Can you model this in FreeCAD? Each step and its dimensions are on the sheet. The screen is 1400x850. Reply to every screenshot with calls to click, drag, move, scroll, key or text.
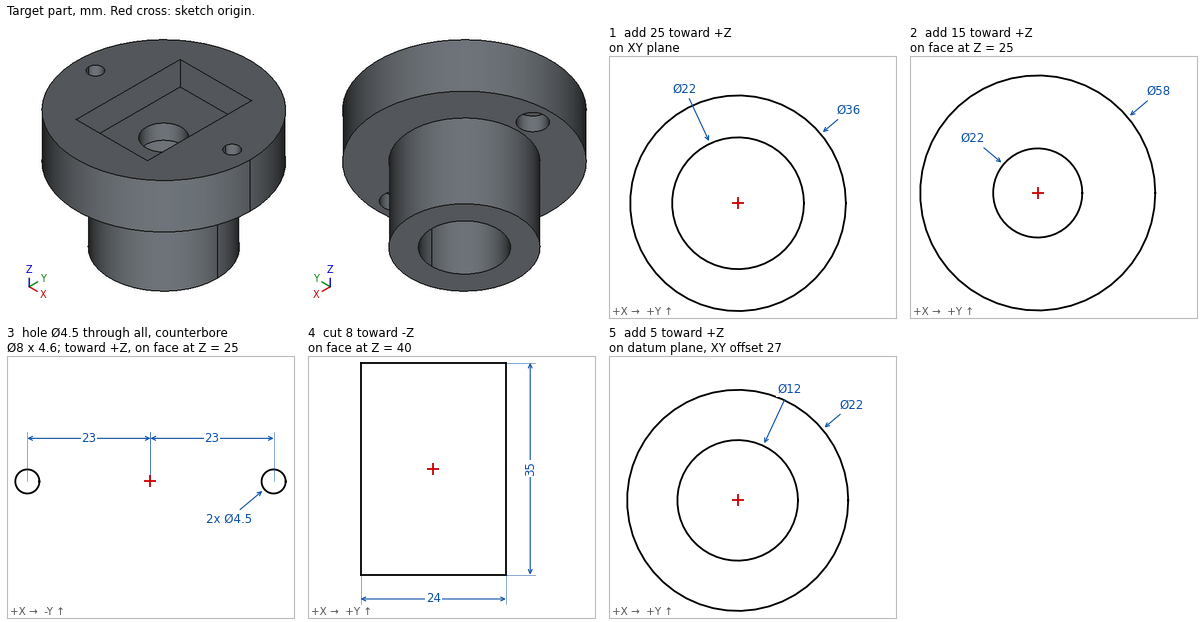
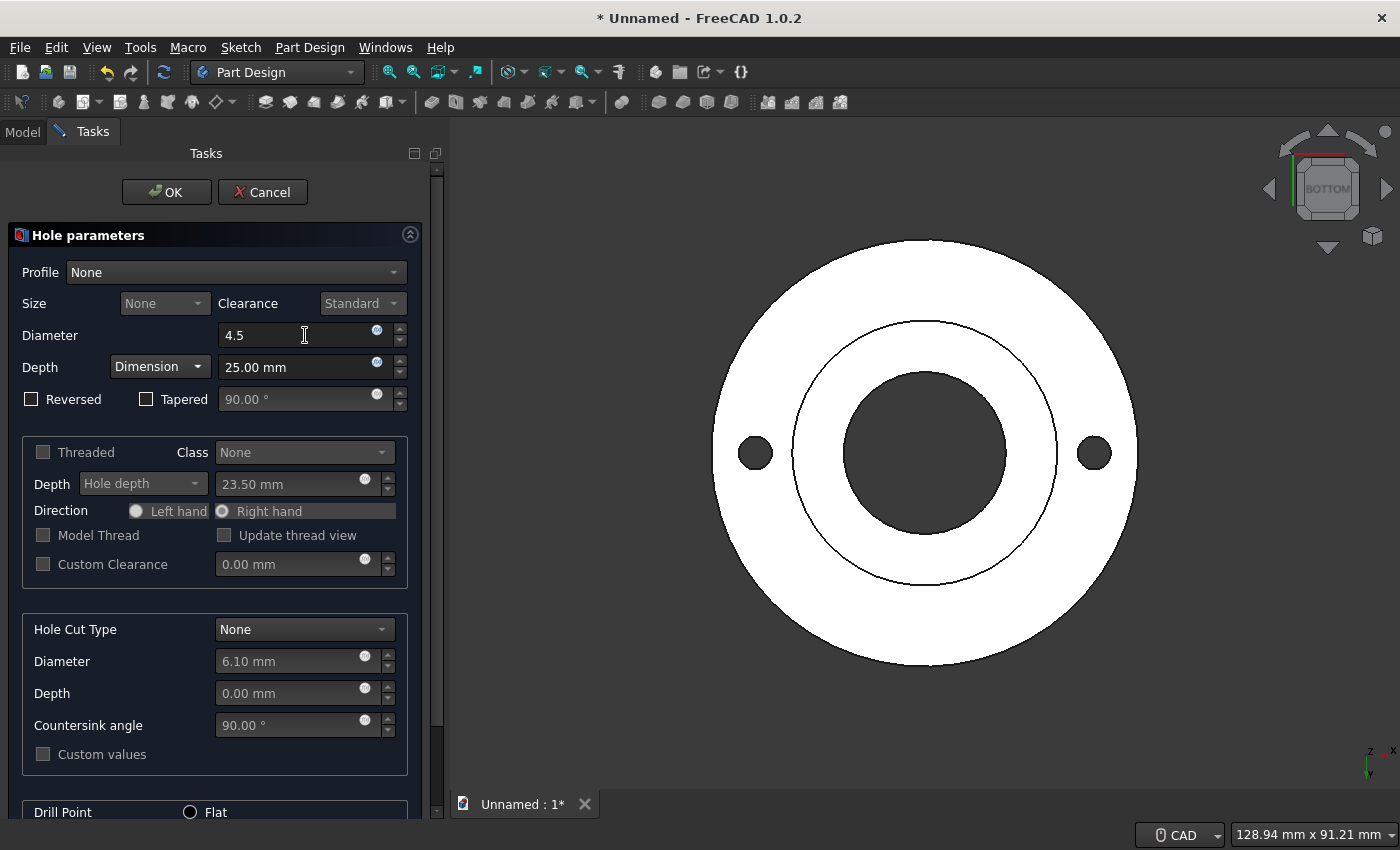
click(161, 366)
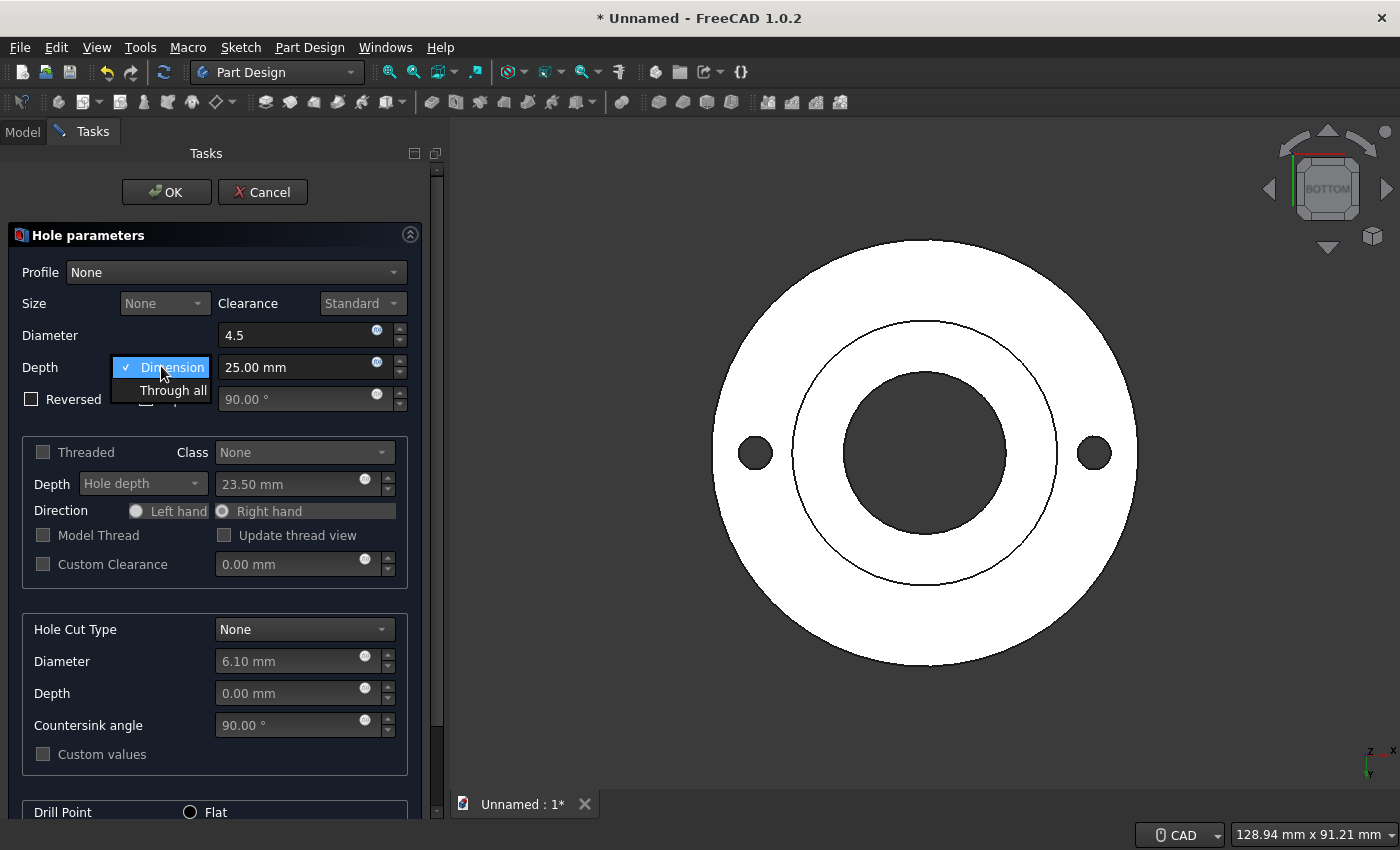
click(160, 390)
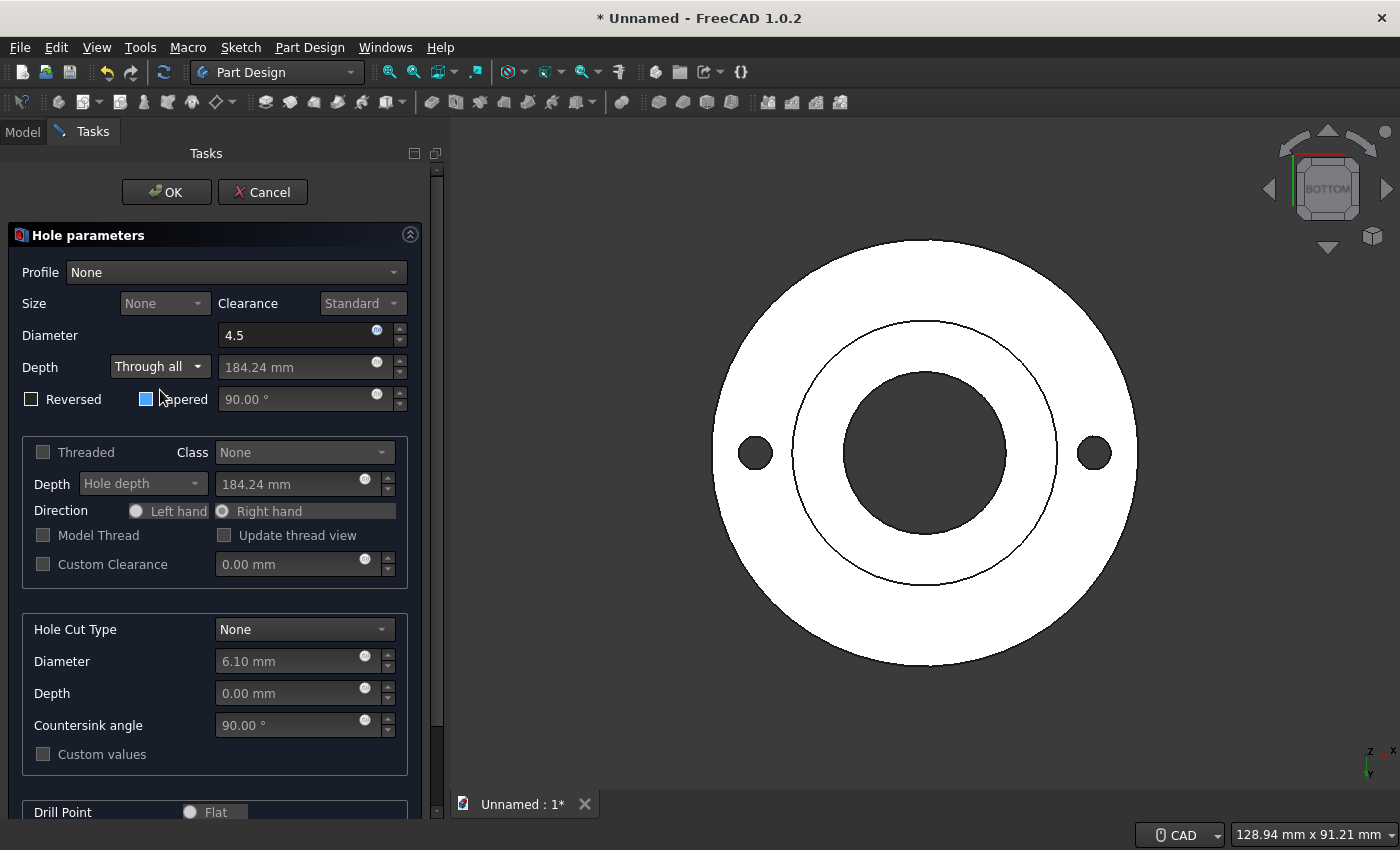
click(306, 630)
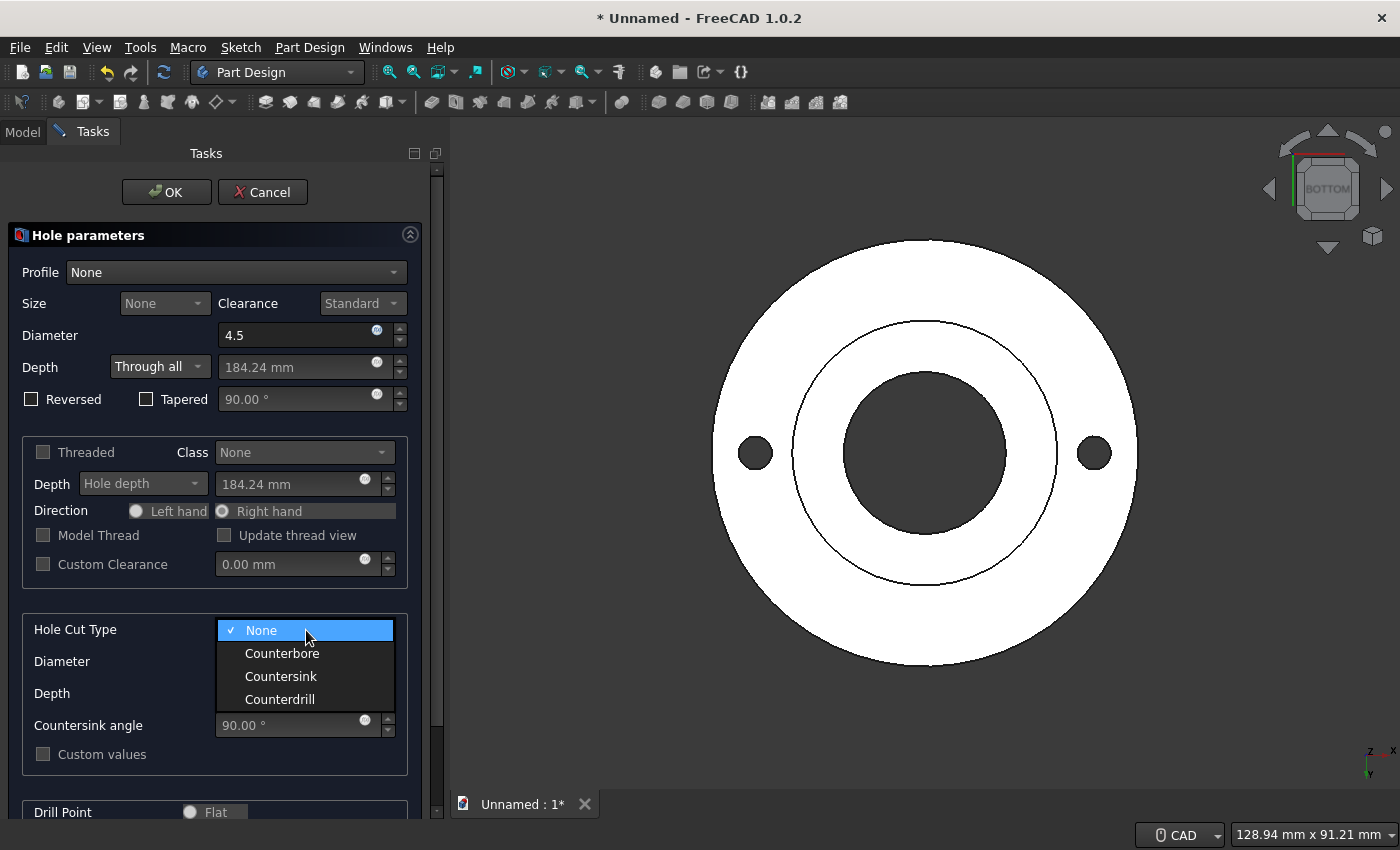
click(304, 654)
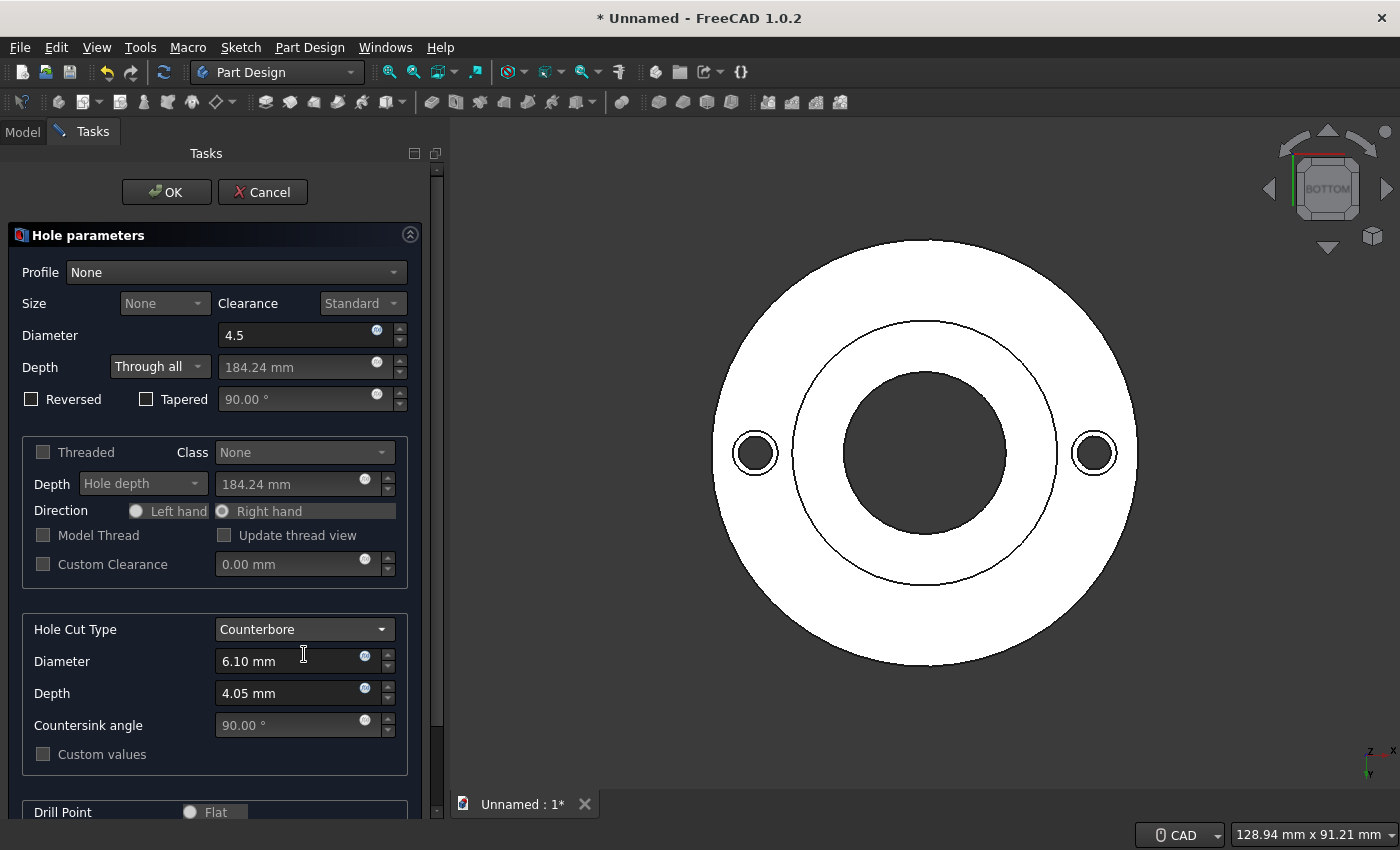
triple_click(298, 661)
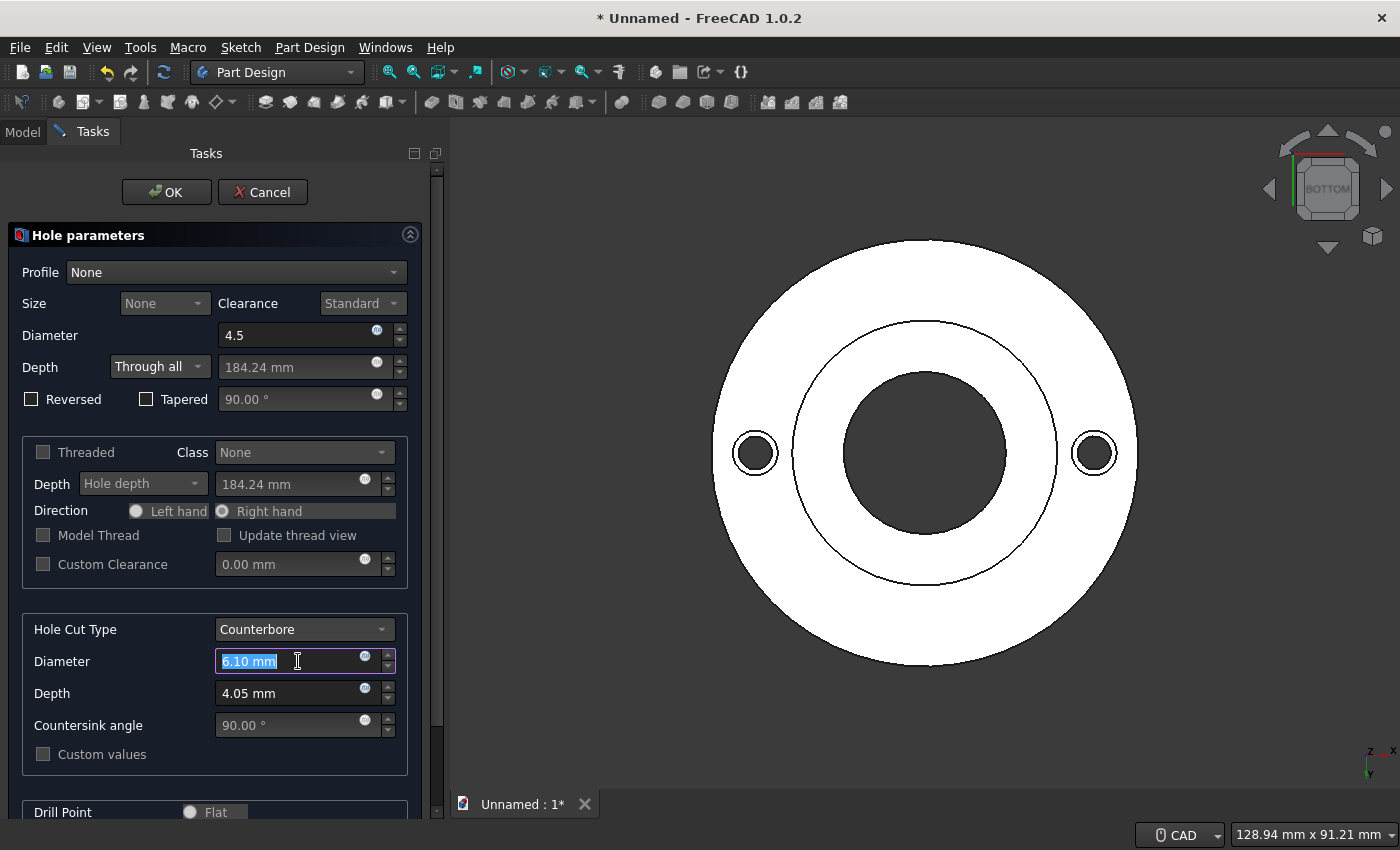
text(8)
key(Tab)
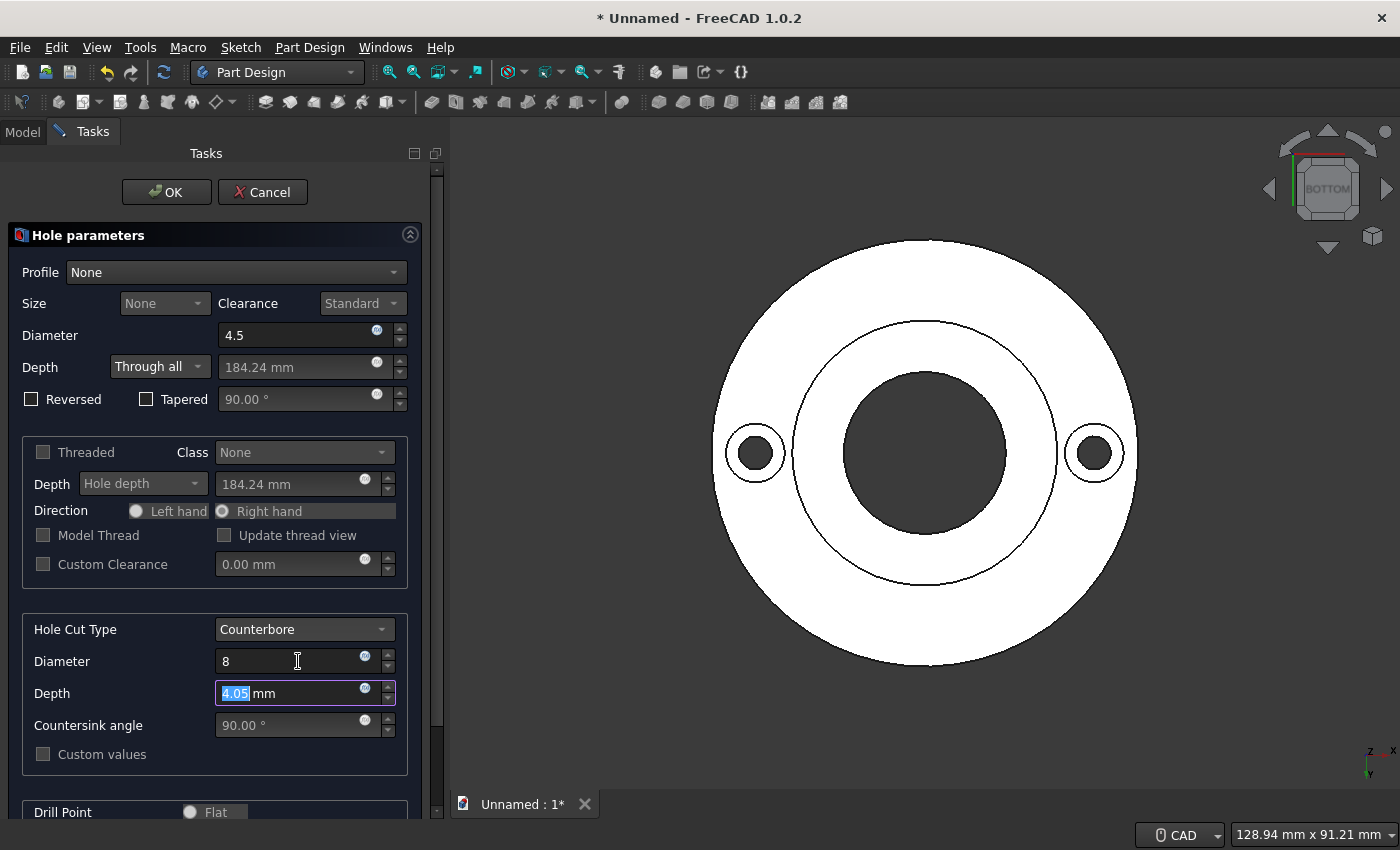
text(4.6)
key(Tab)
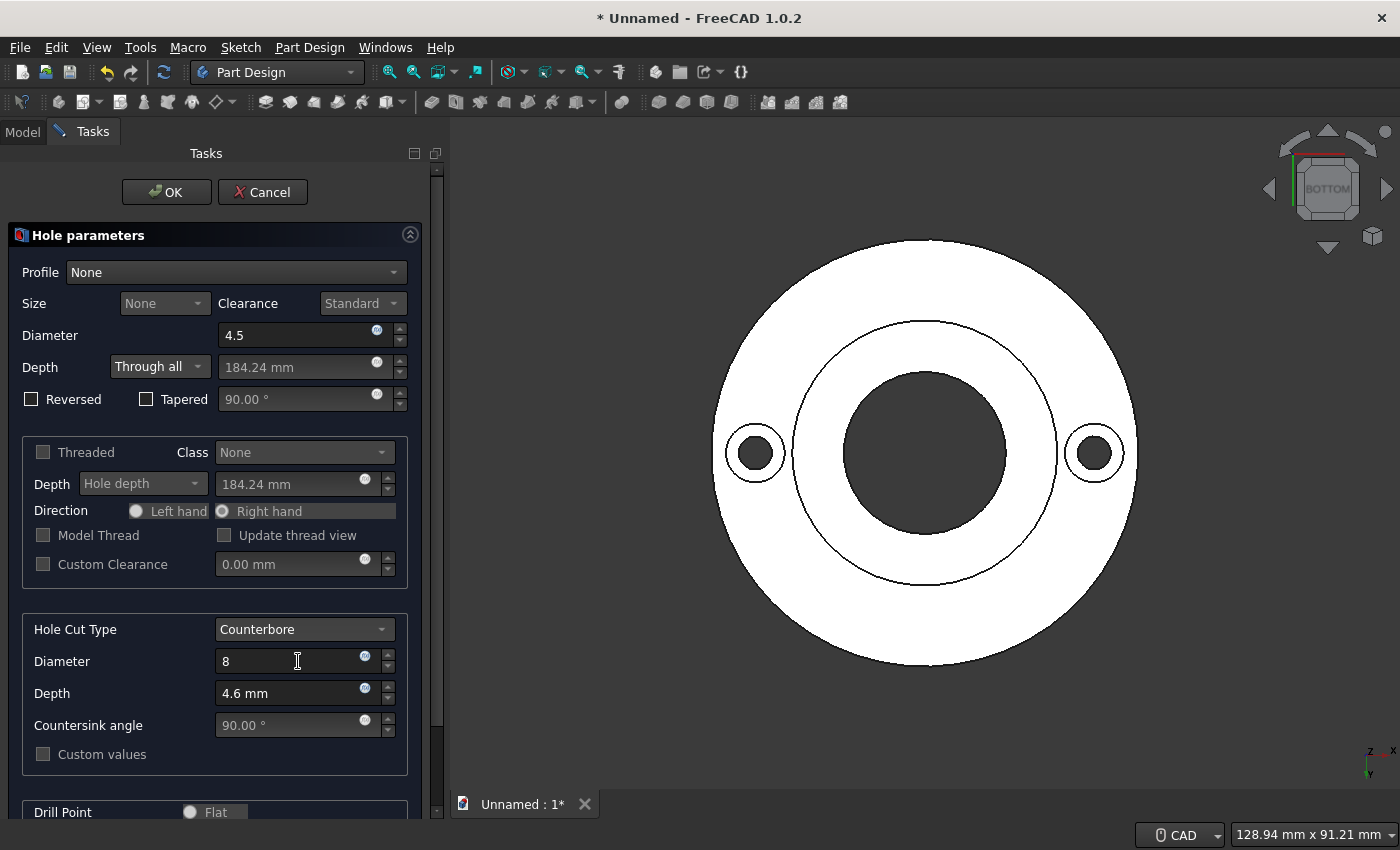
click(167, 192)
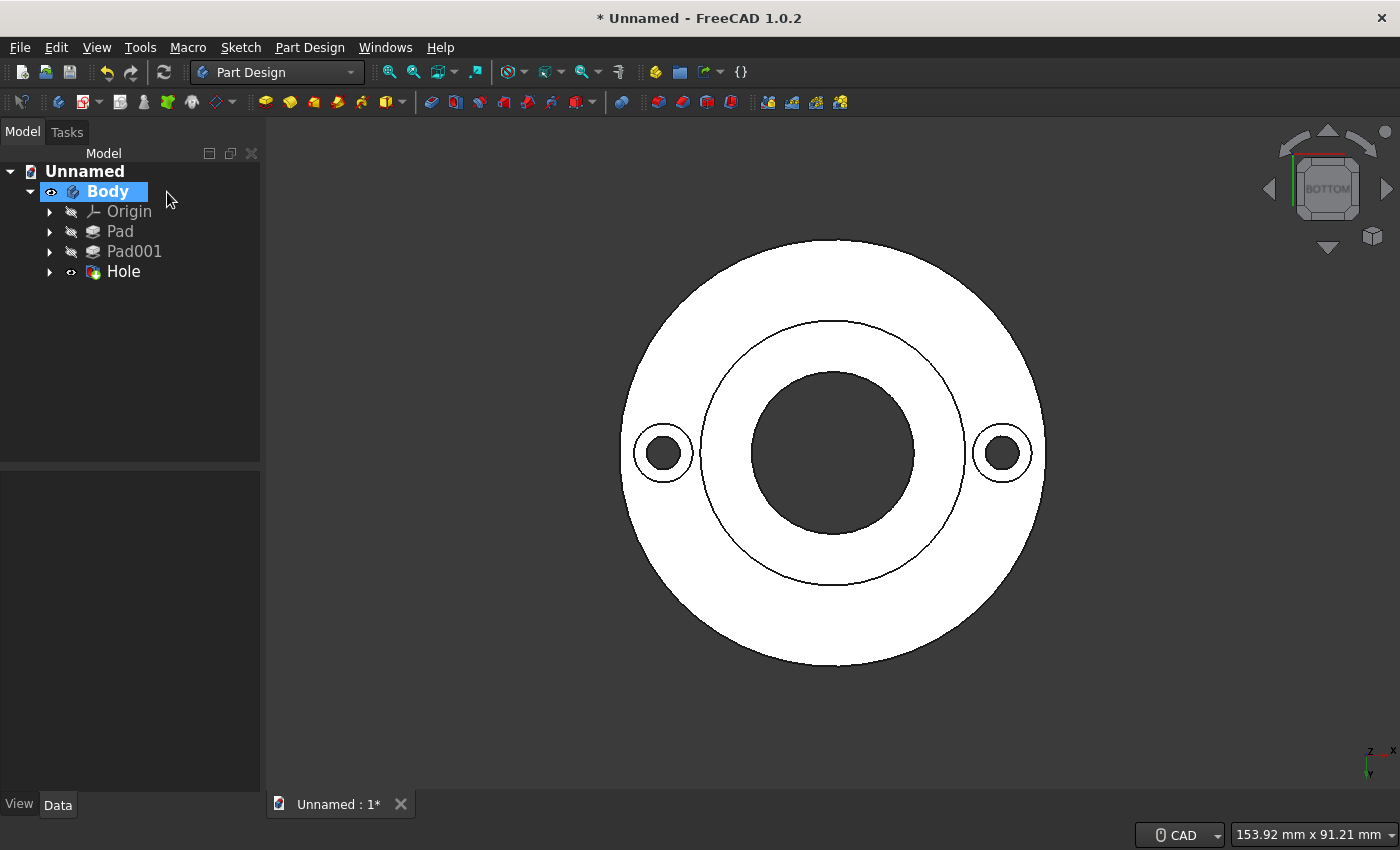
key(0)